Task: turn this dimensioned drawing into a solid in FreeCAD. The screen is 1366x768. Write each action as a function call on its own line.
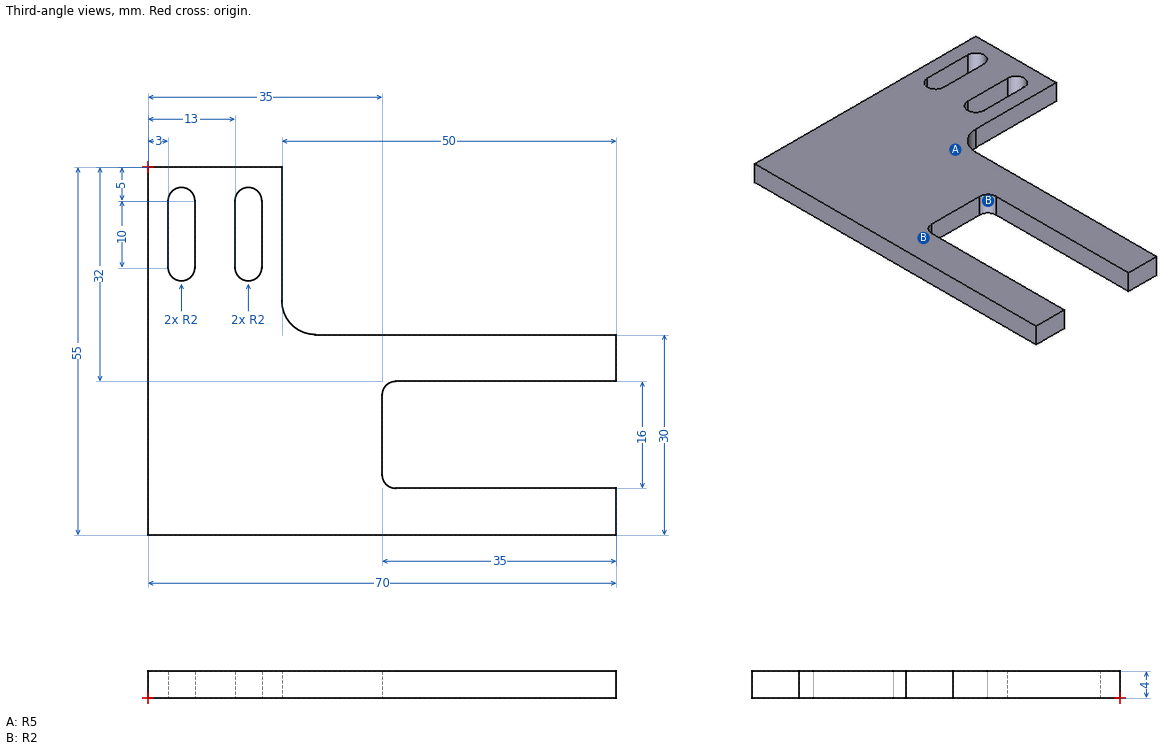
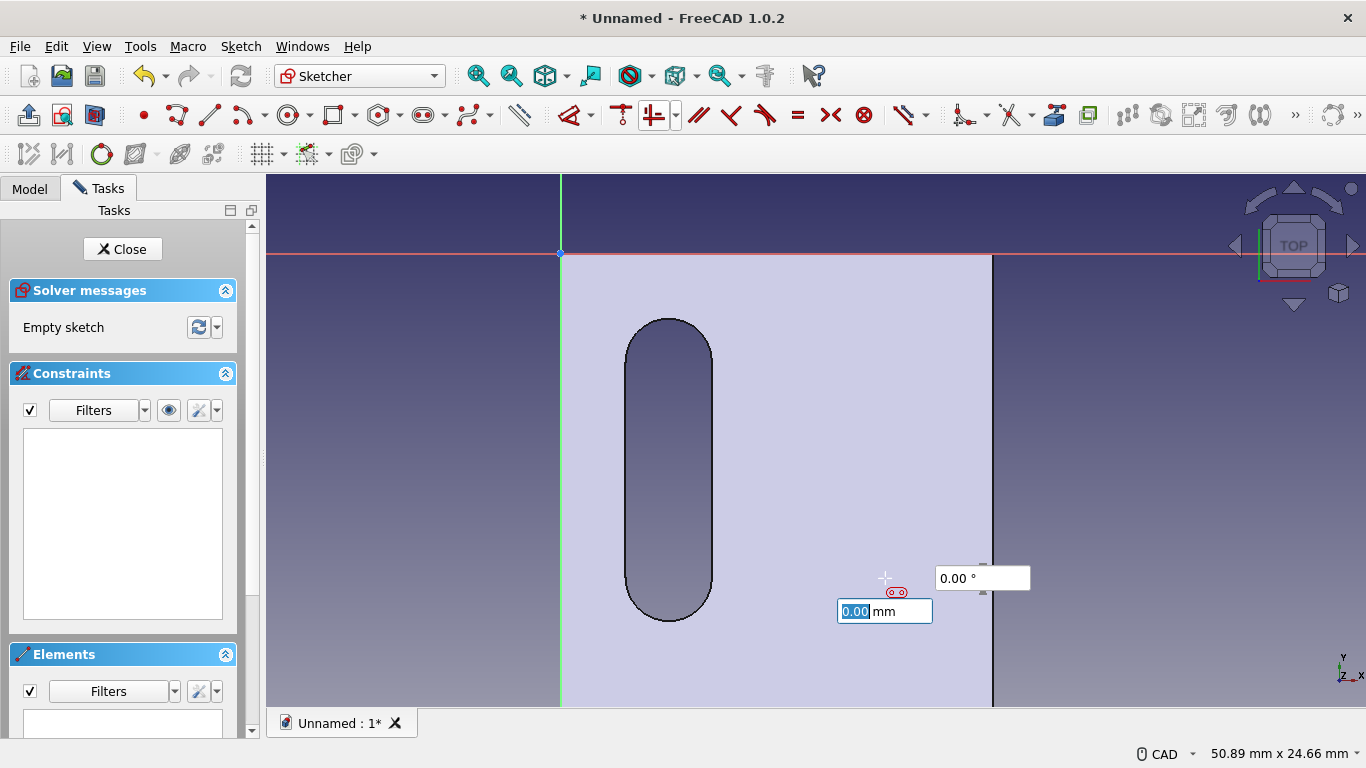
click(885, 362)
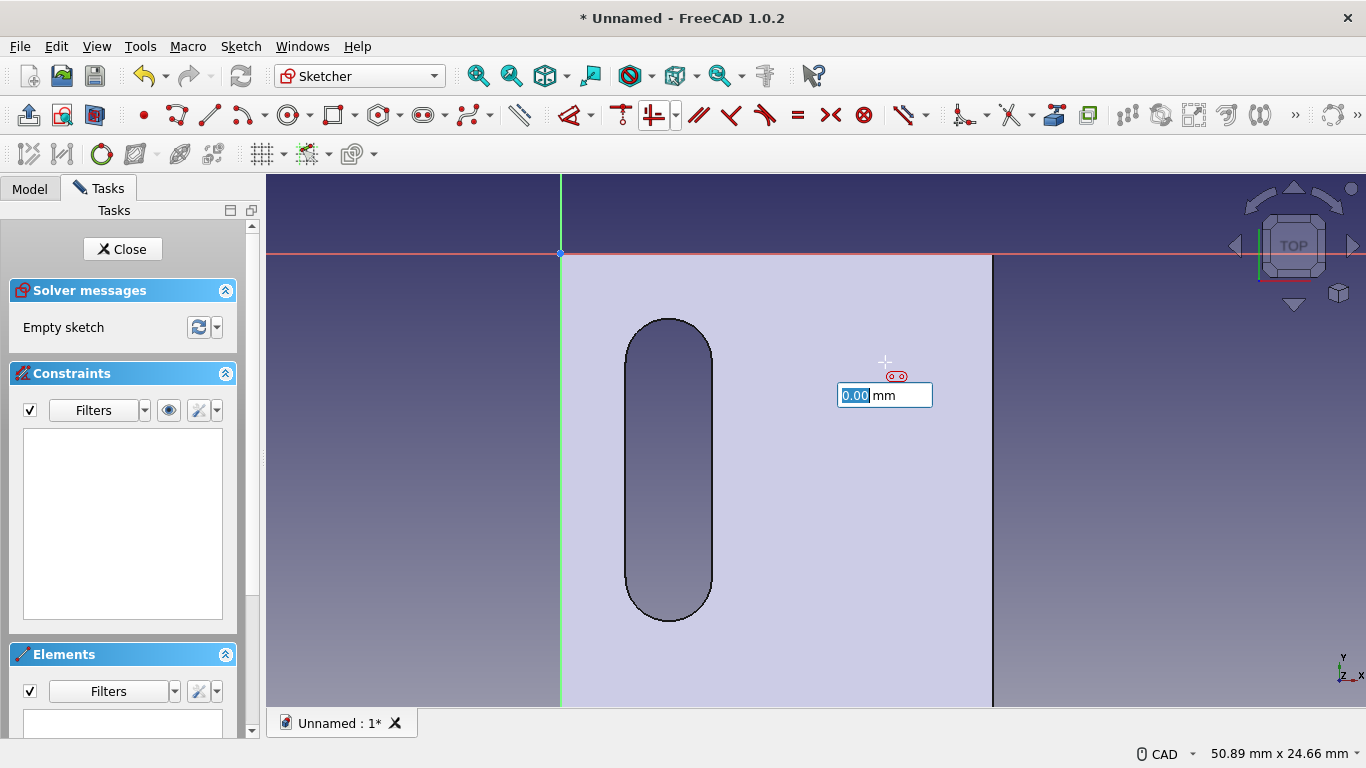
click(842, 470)
key(Escape)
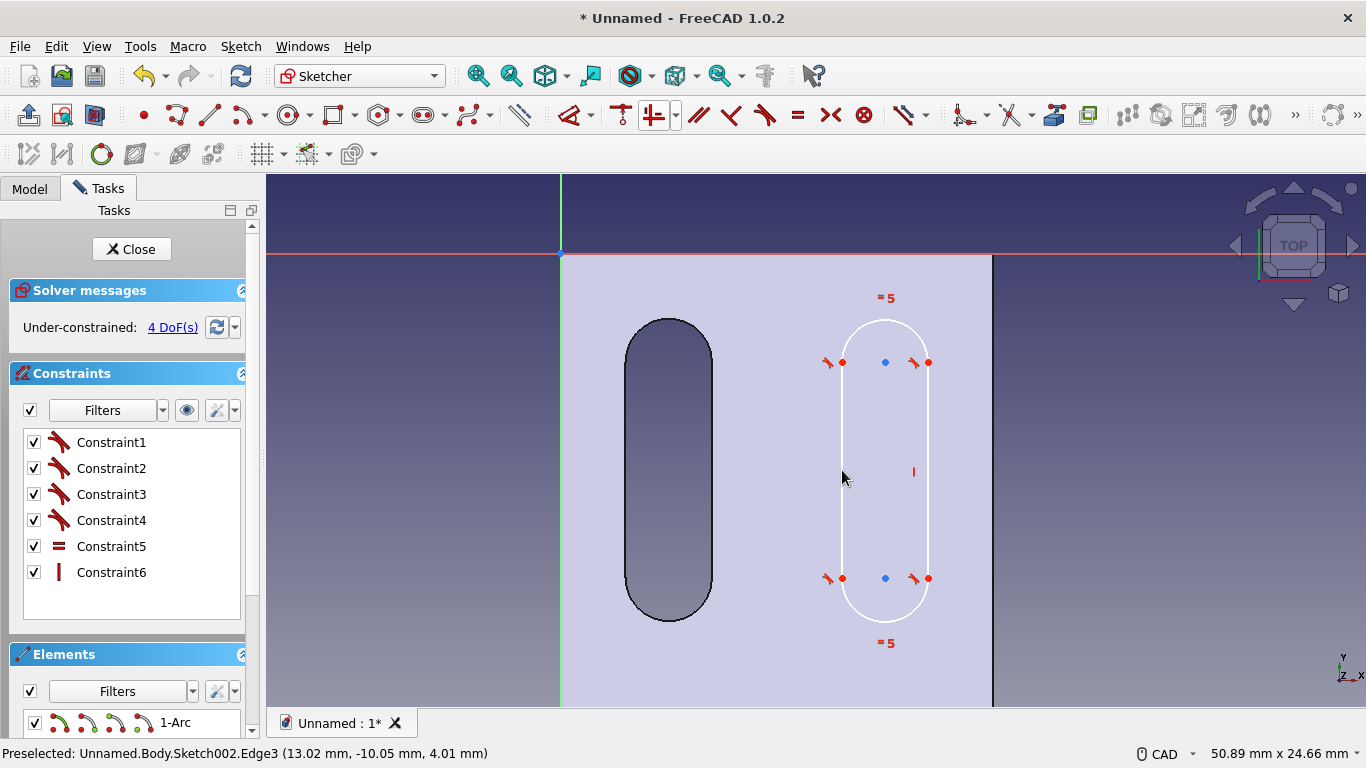
click(568, 116)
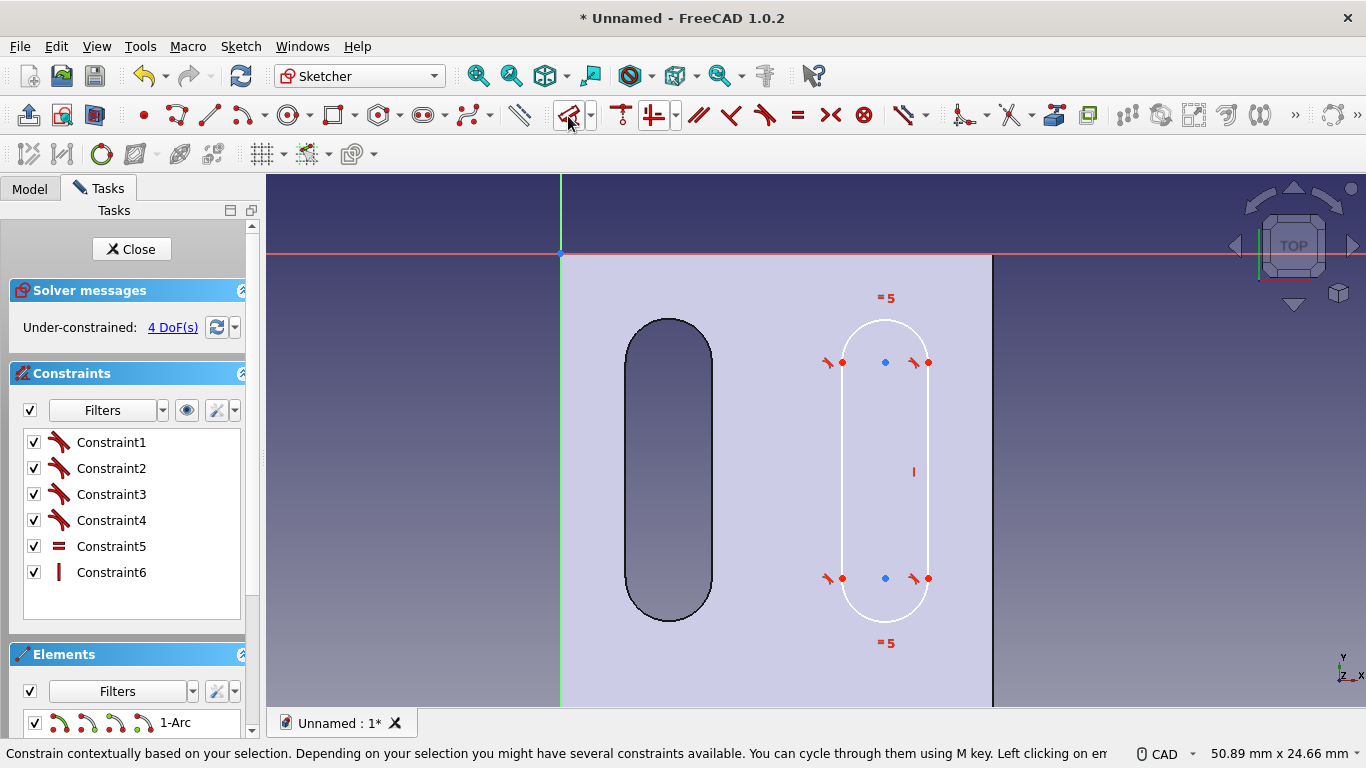
click(860, 614)
click(841, 640)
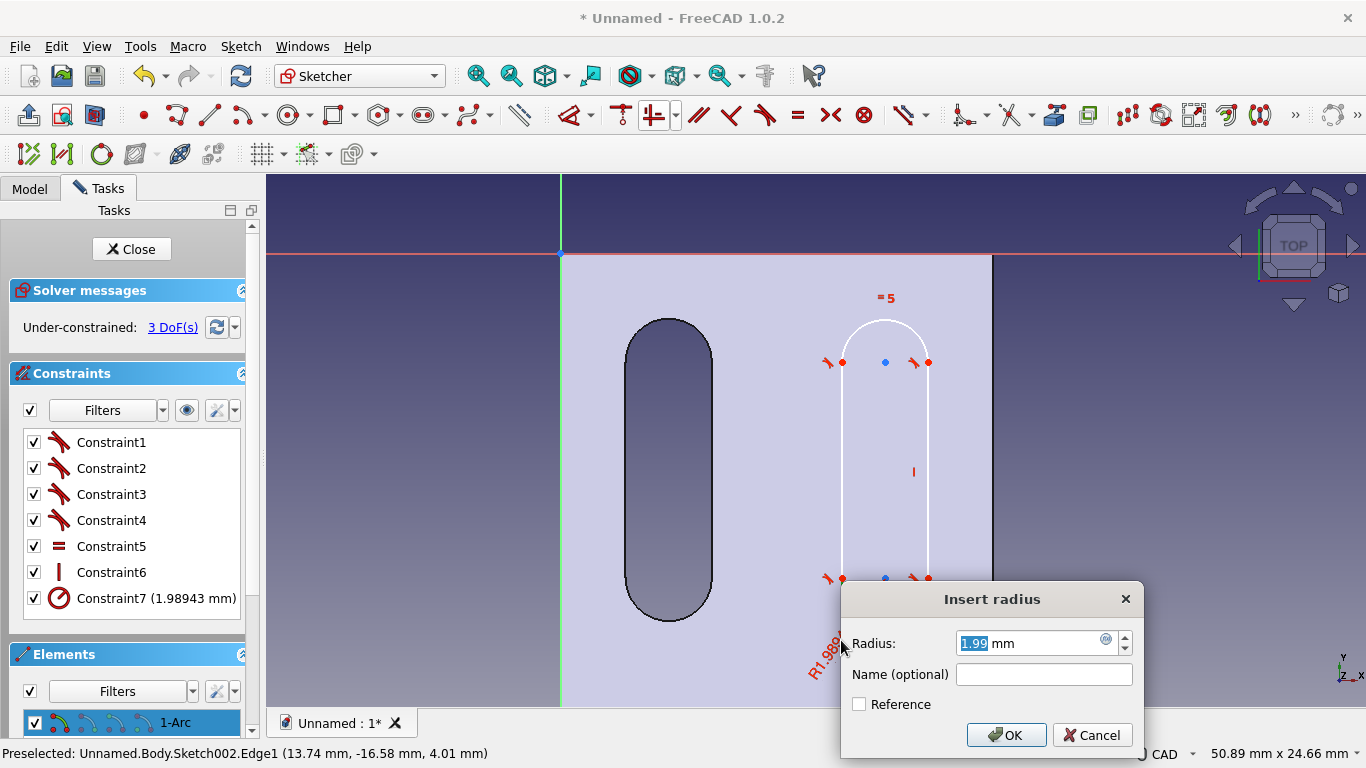
text(2)
key(Return)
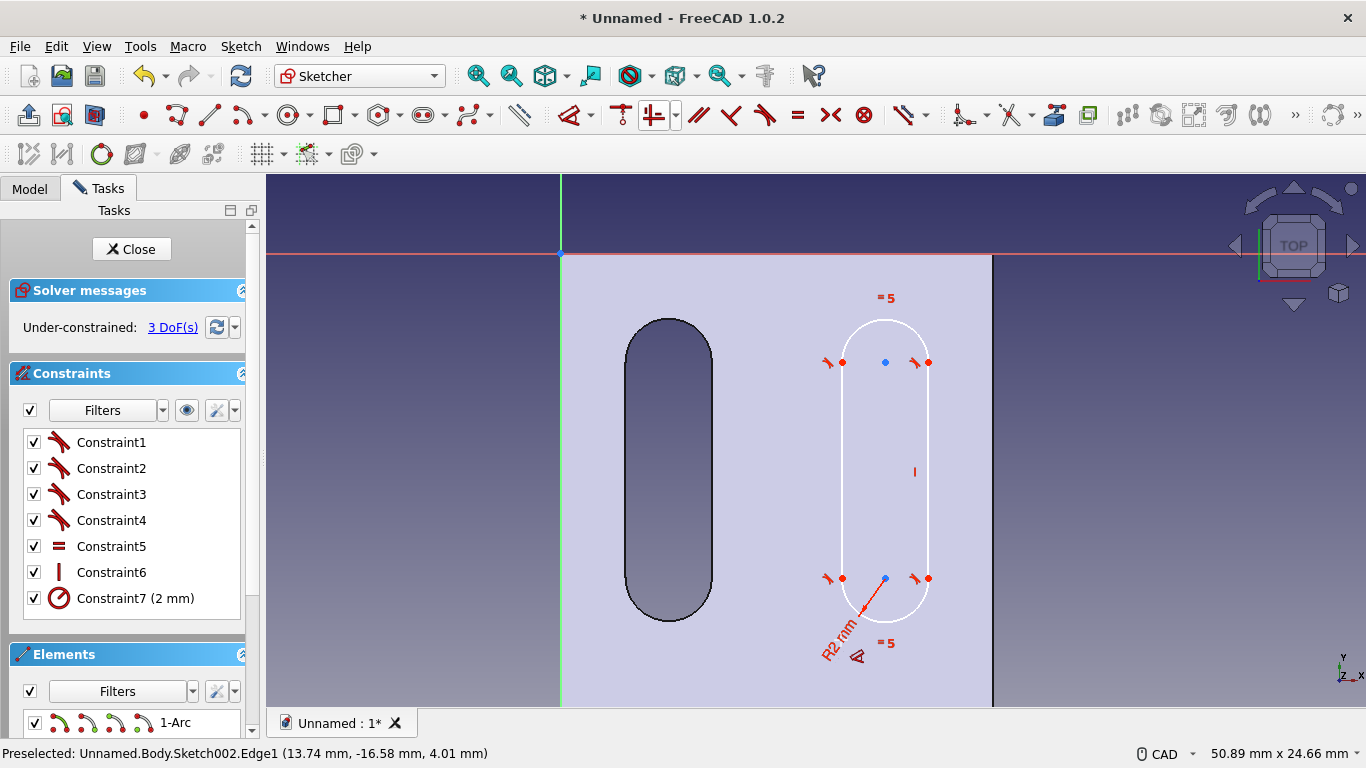
click(842, 514)
click(876, 471)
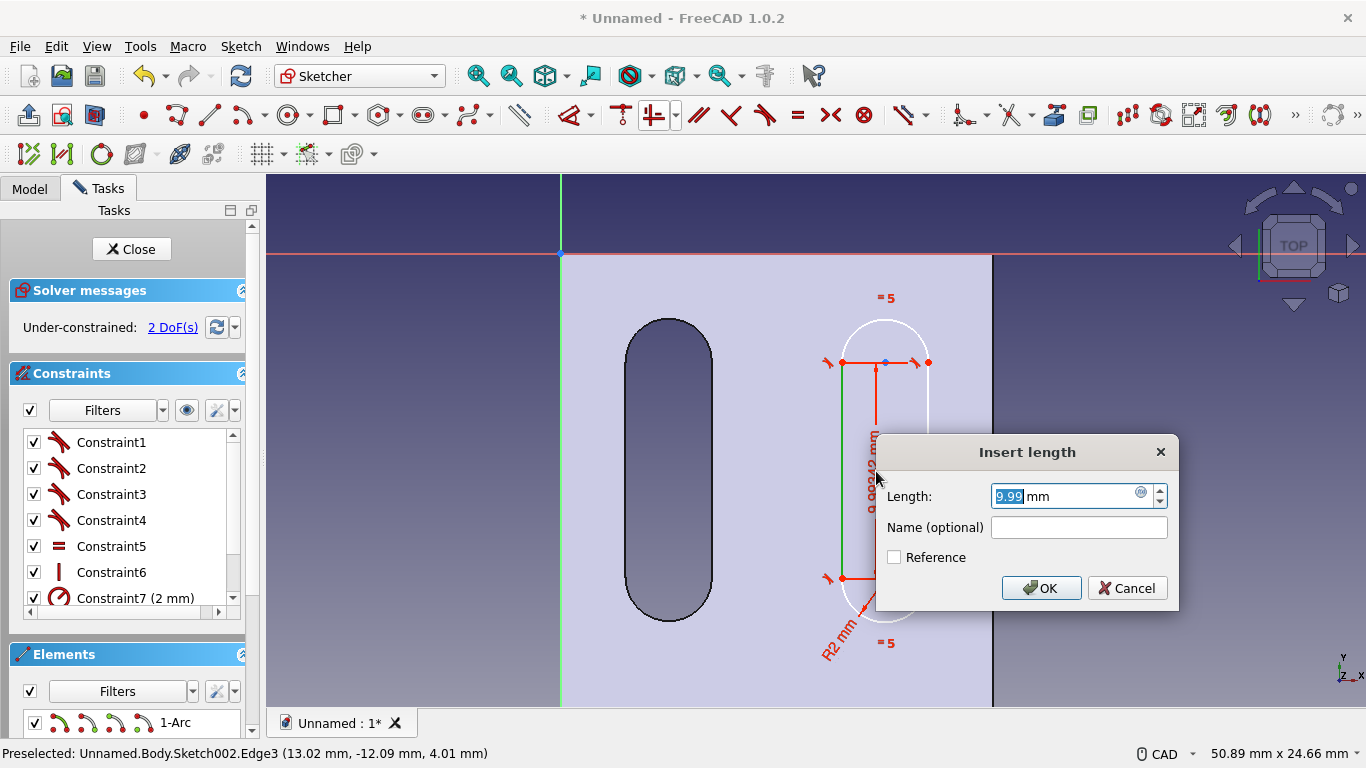
text(10)
key(Return)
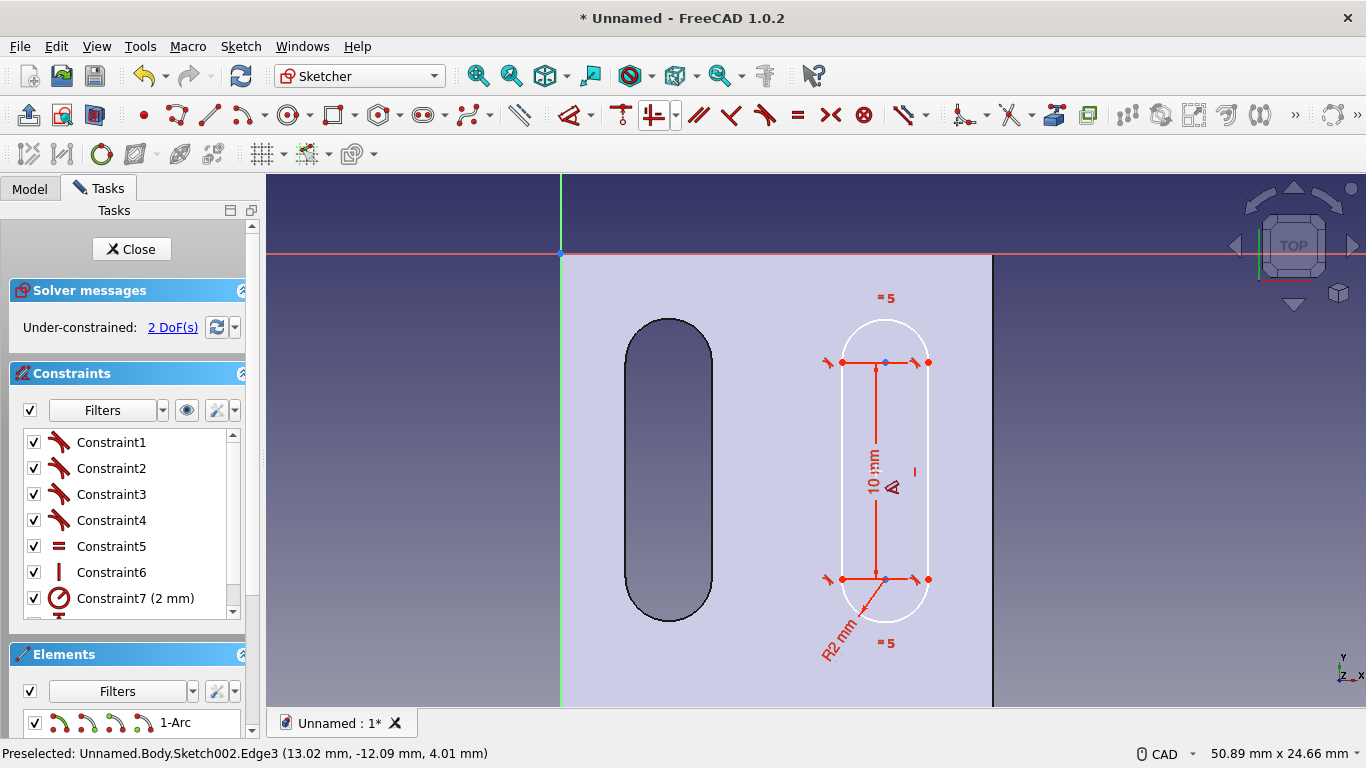
click(928, 363)
click(962, 308)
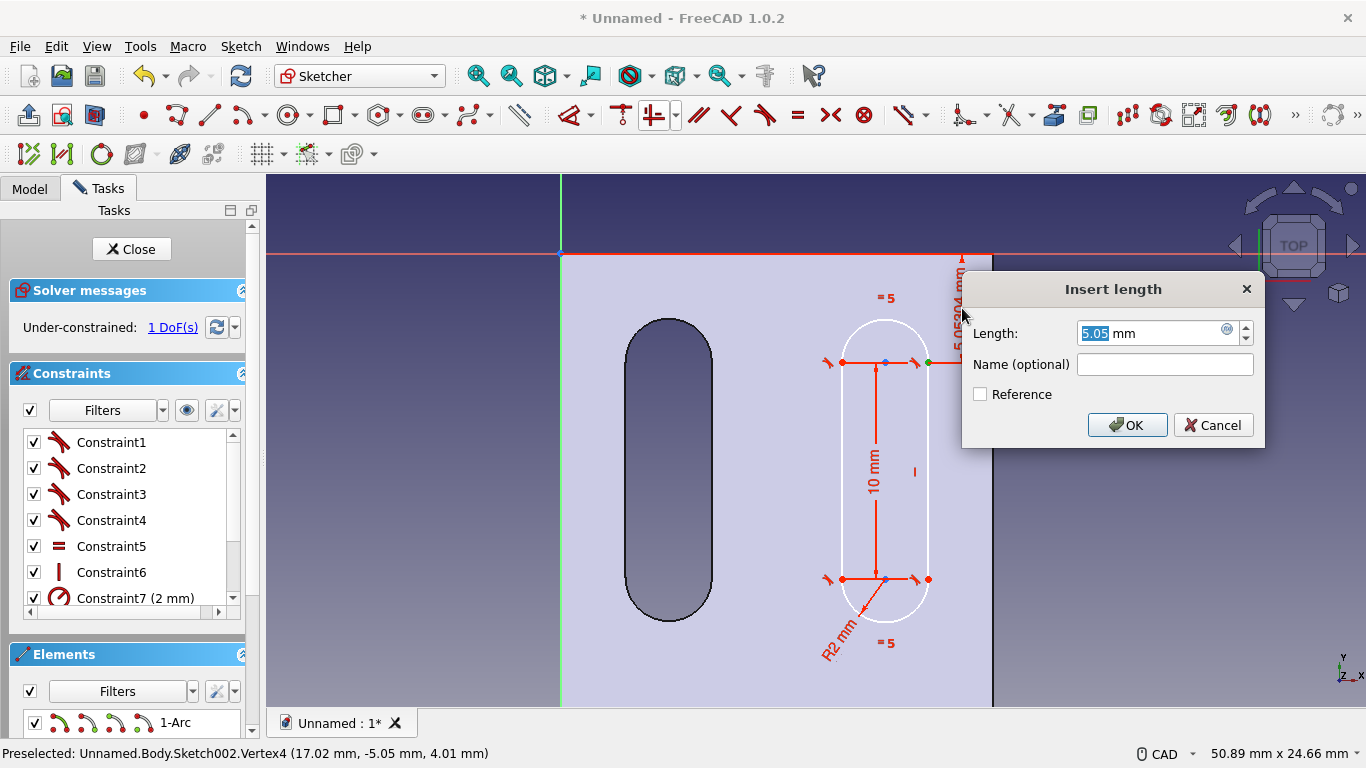
text(5)
key(Return)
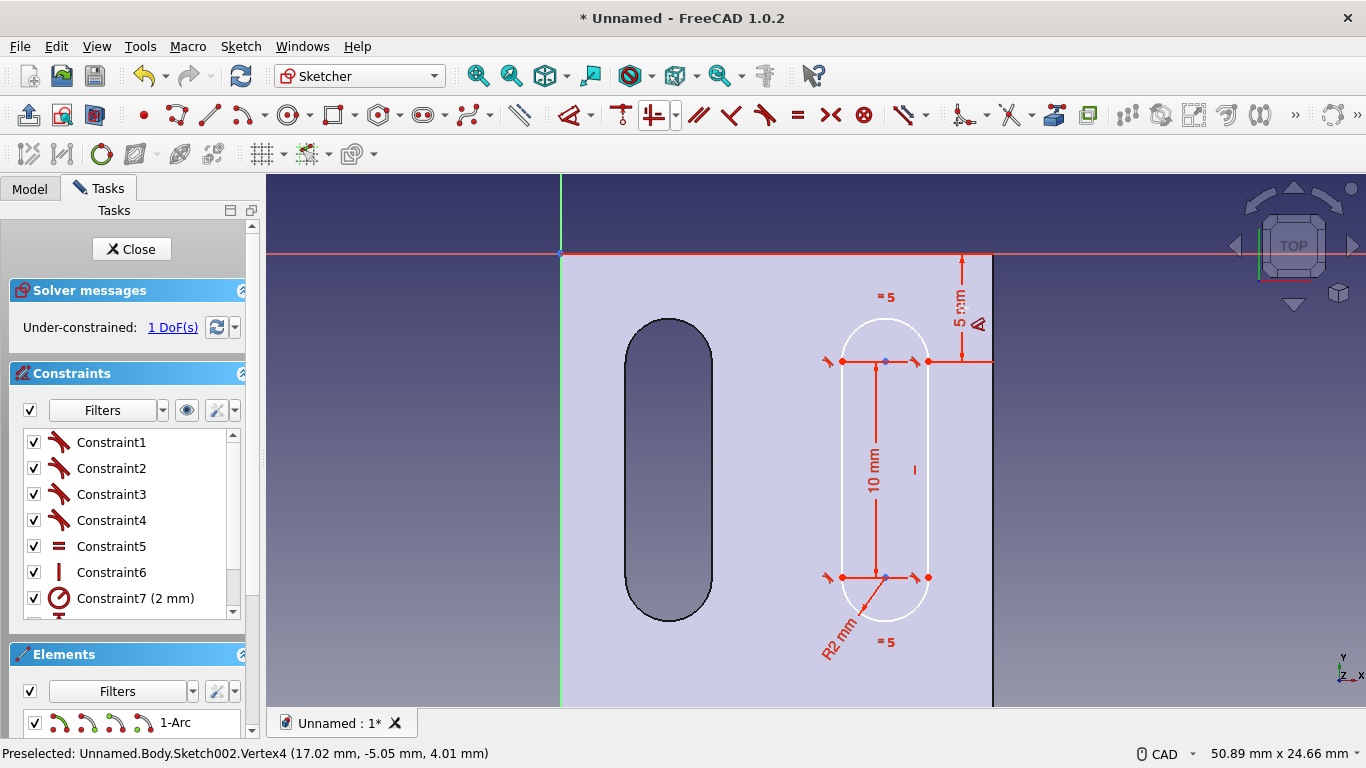
click(842, 578)
click(701, 220)